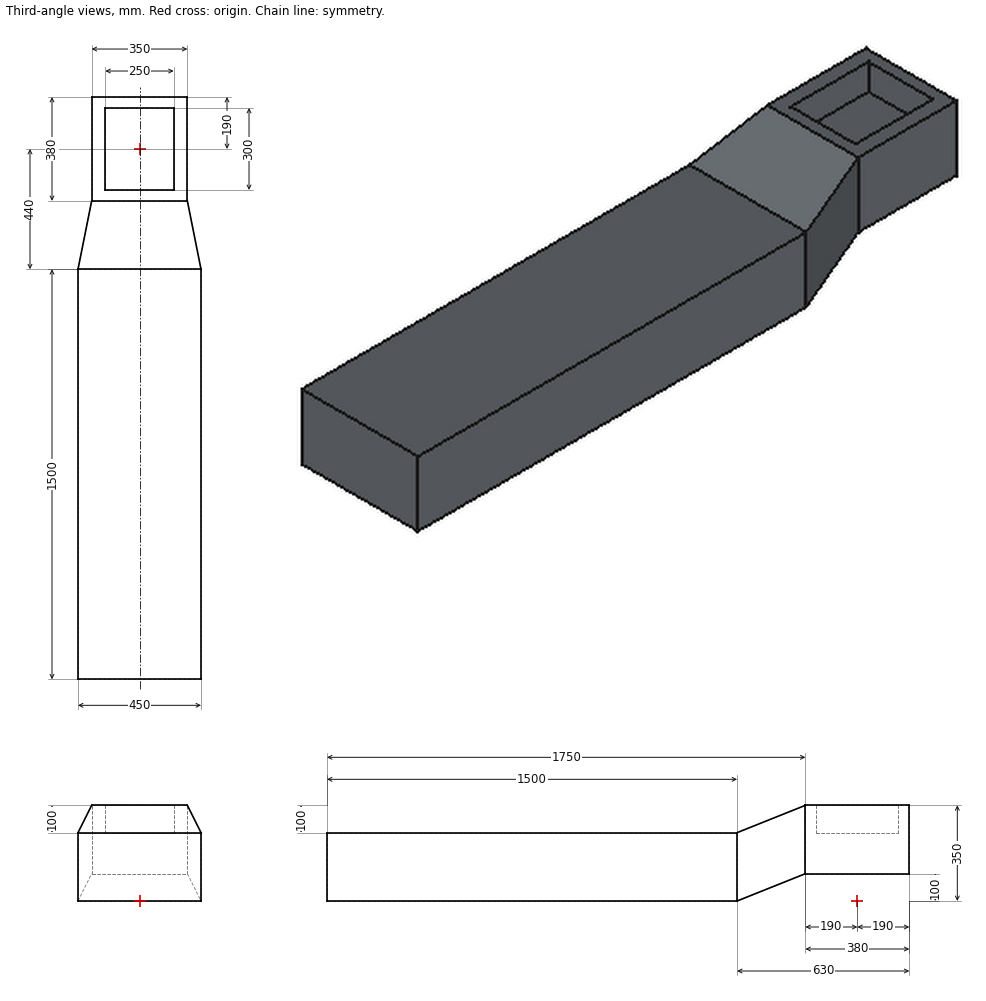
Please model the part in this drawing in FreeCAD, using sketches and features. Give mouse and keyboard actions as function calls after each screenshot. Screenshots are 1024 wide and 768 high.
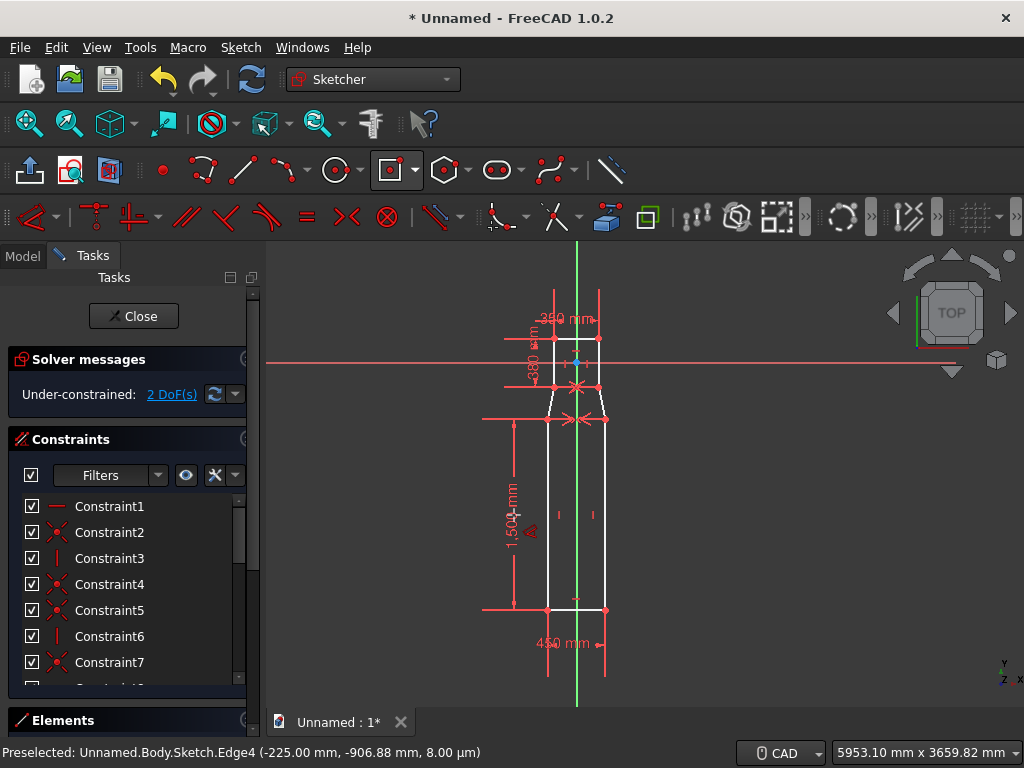
scroll(599, 339, up, 3)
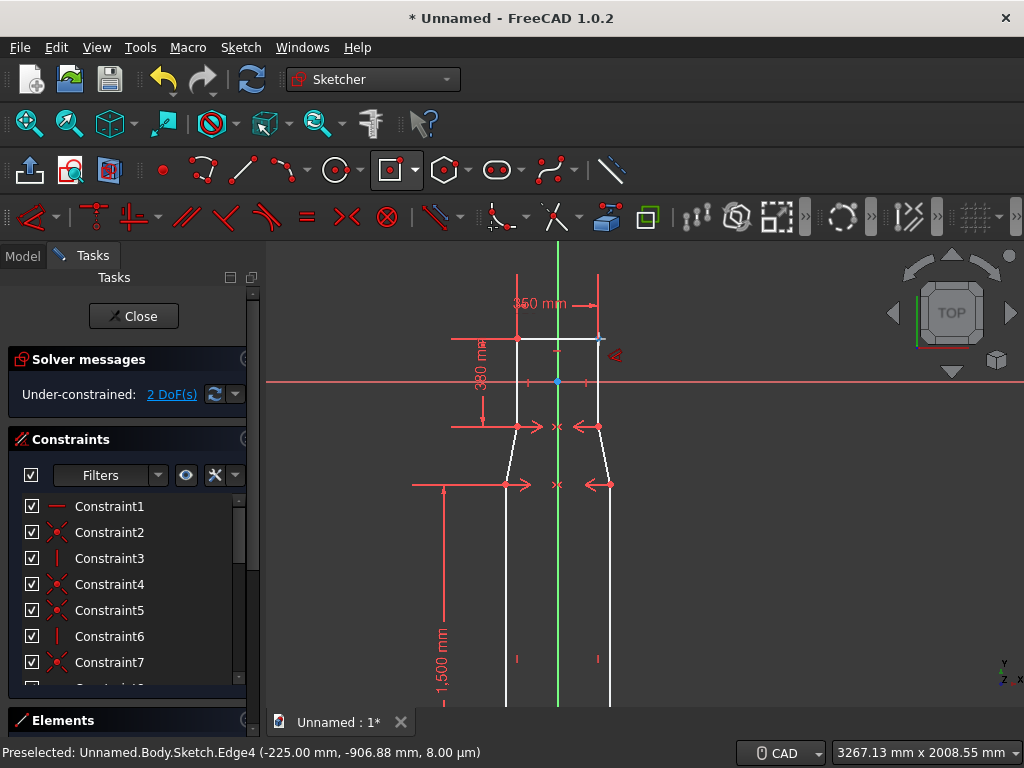
click(598, 339)
click(632, 360)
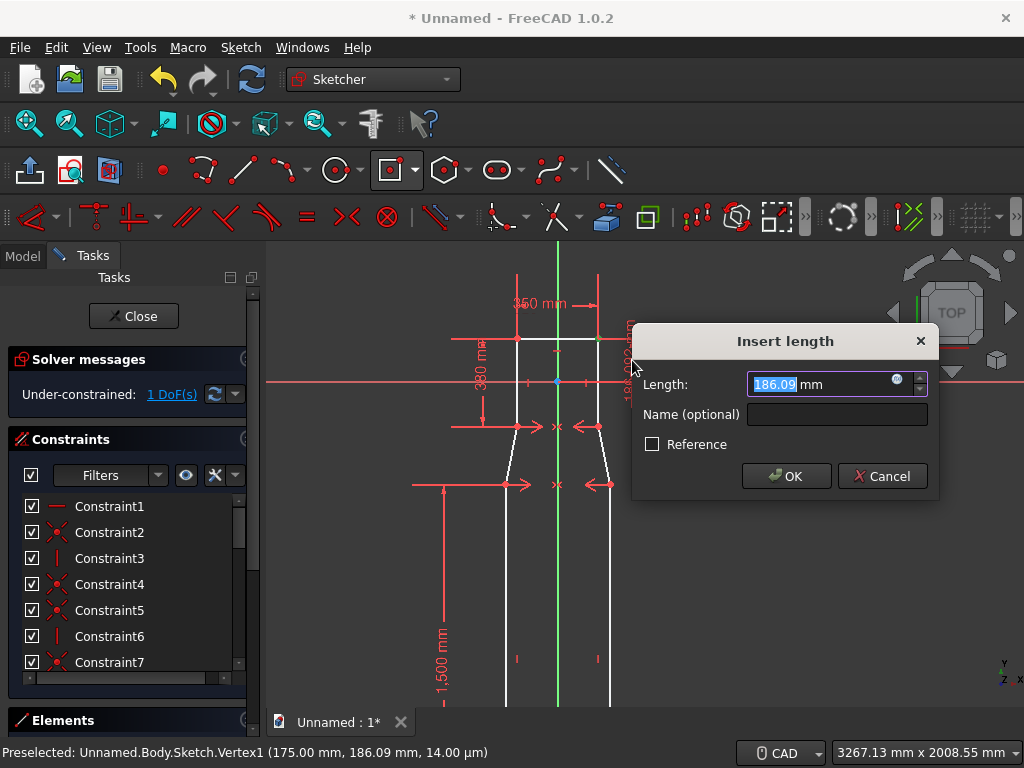
text(190)
key(Return)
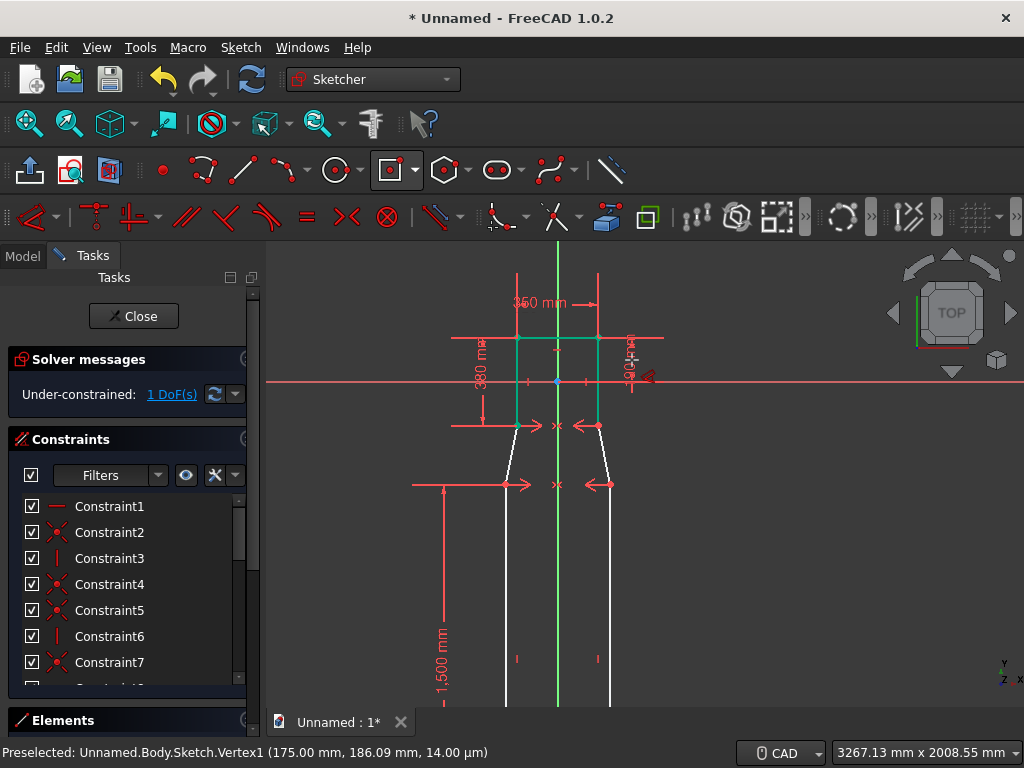
click(506, 485)
click(472, 433)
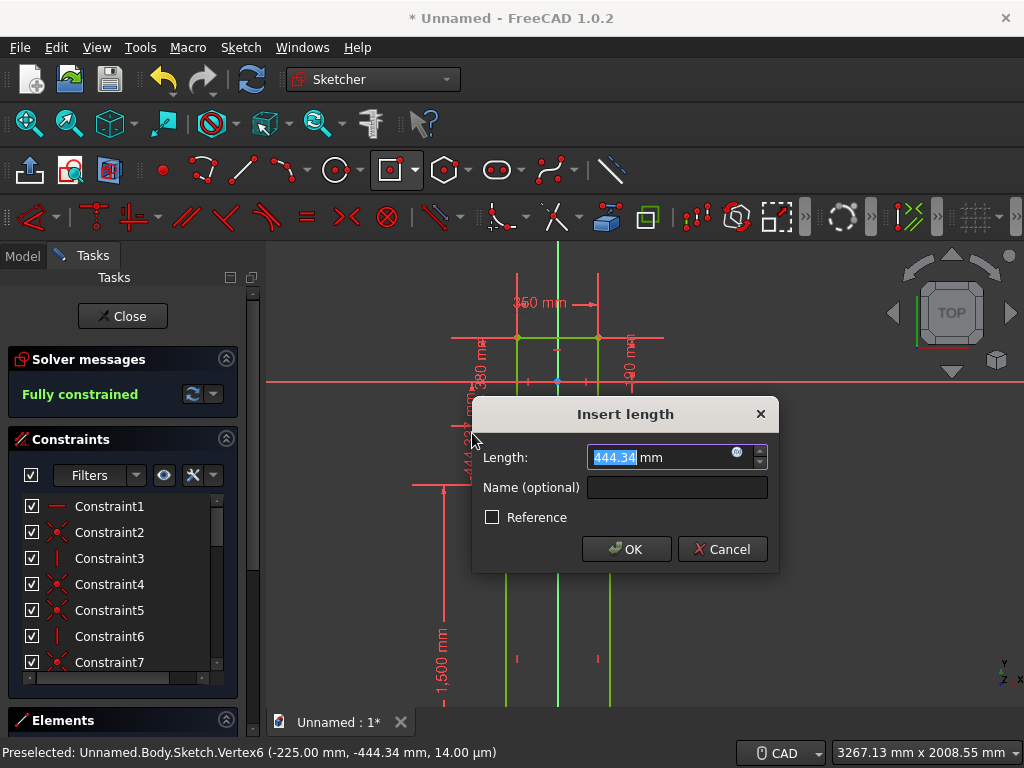
text(440)
key(Return)
key(Escape)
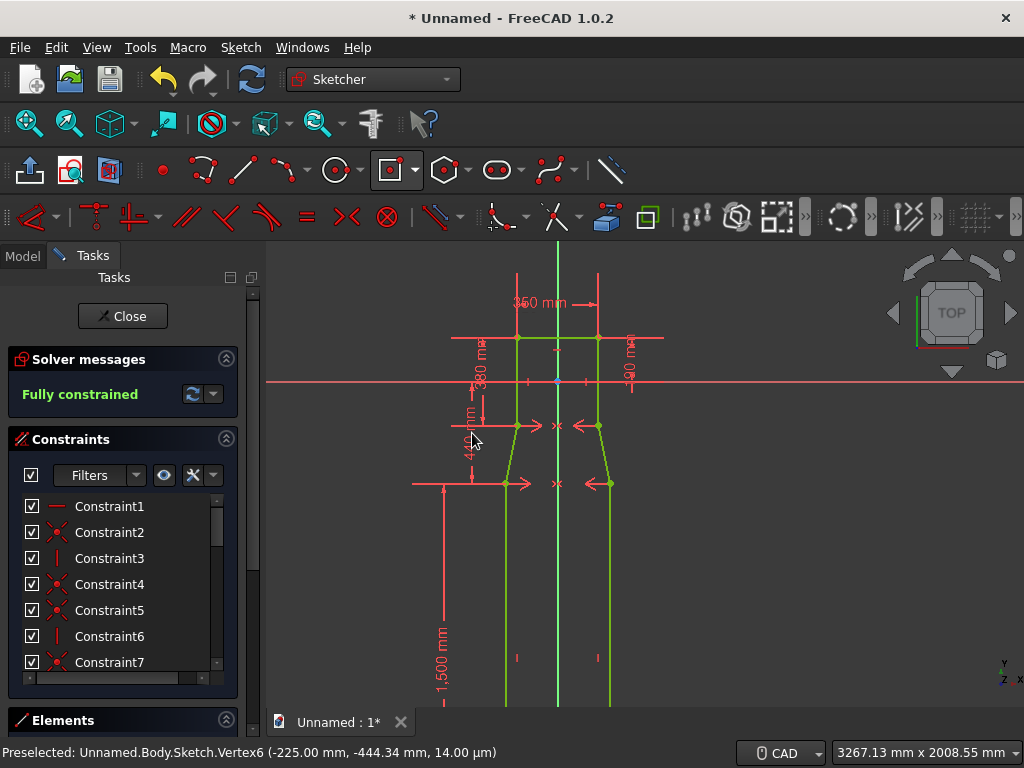
click(123, 316)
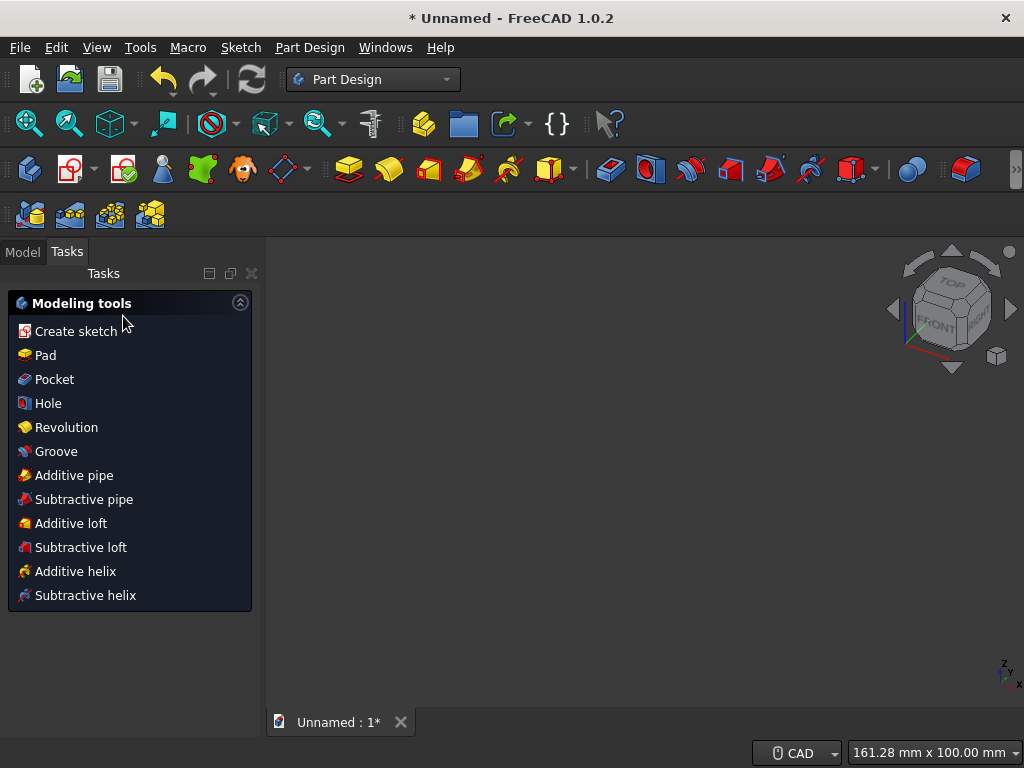
click(350, 170)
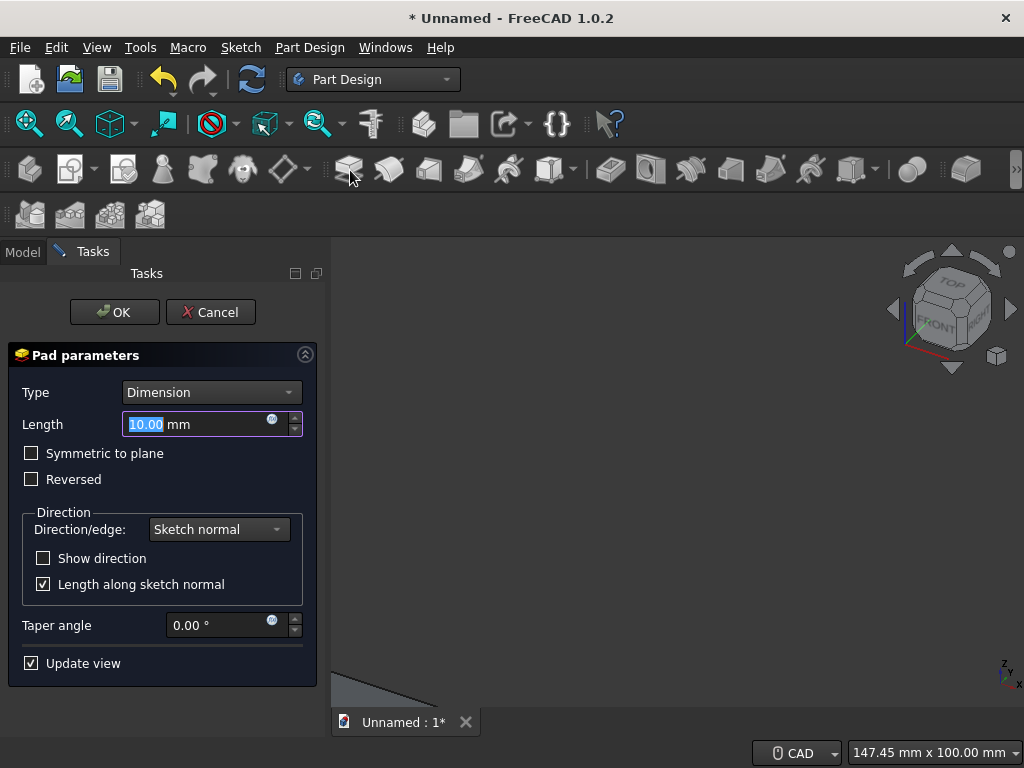
text(350)
key(Tab)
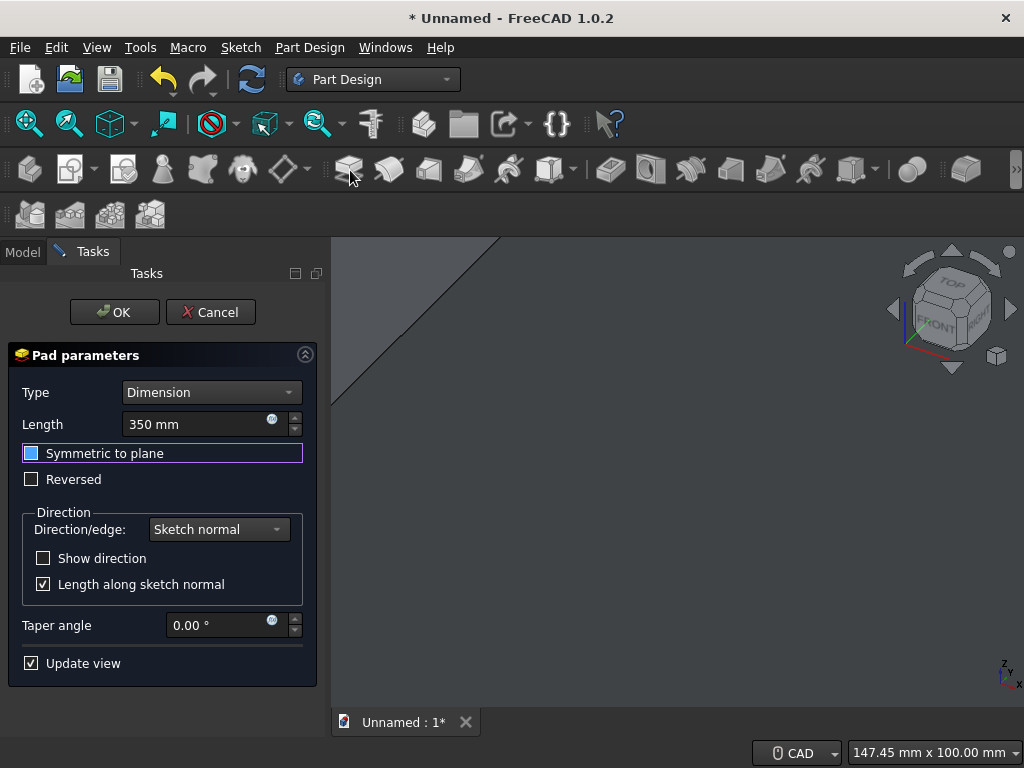
click(115, 312)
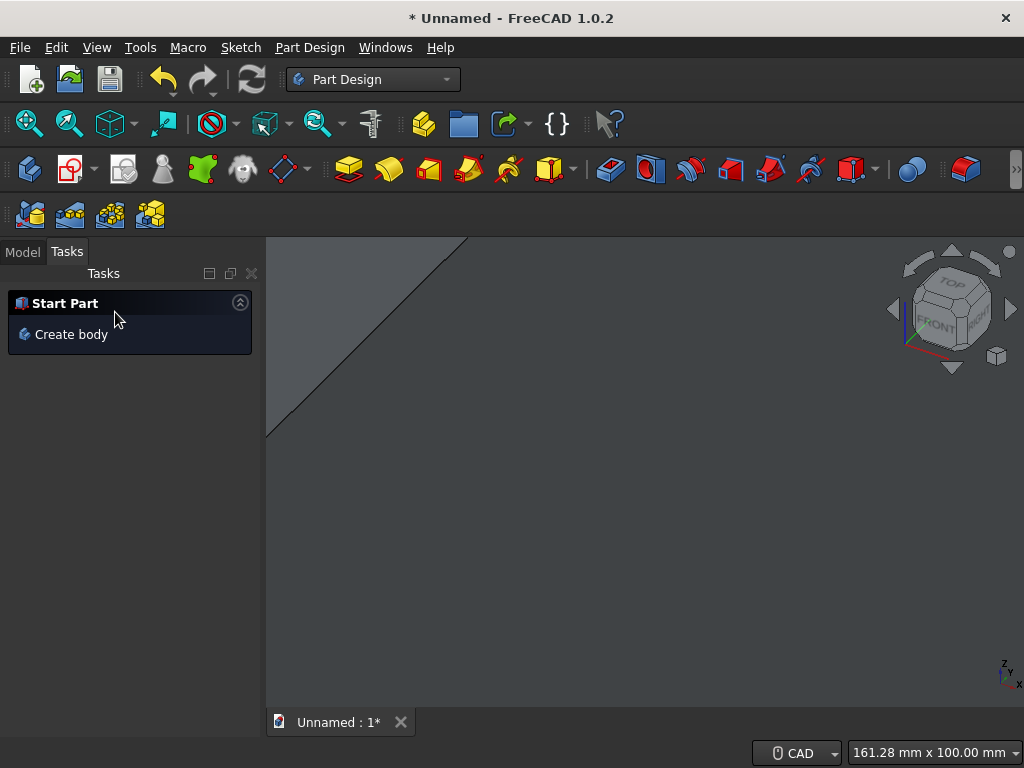
click(30, 124)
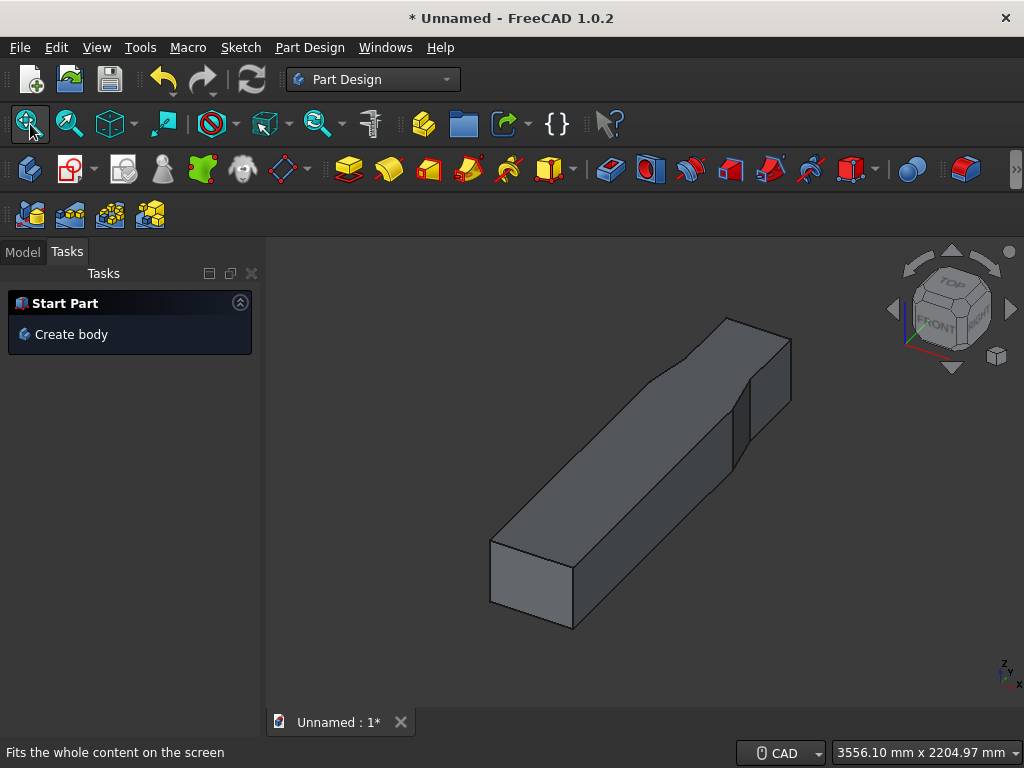
key(6)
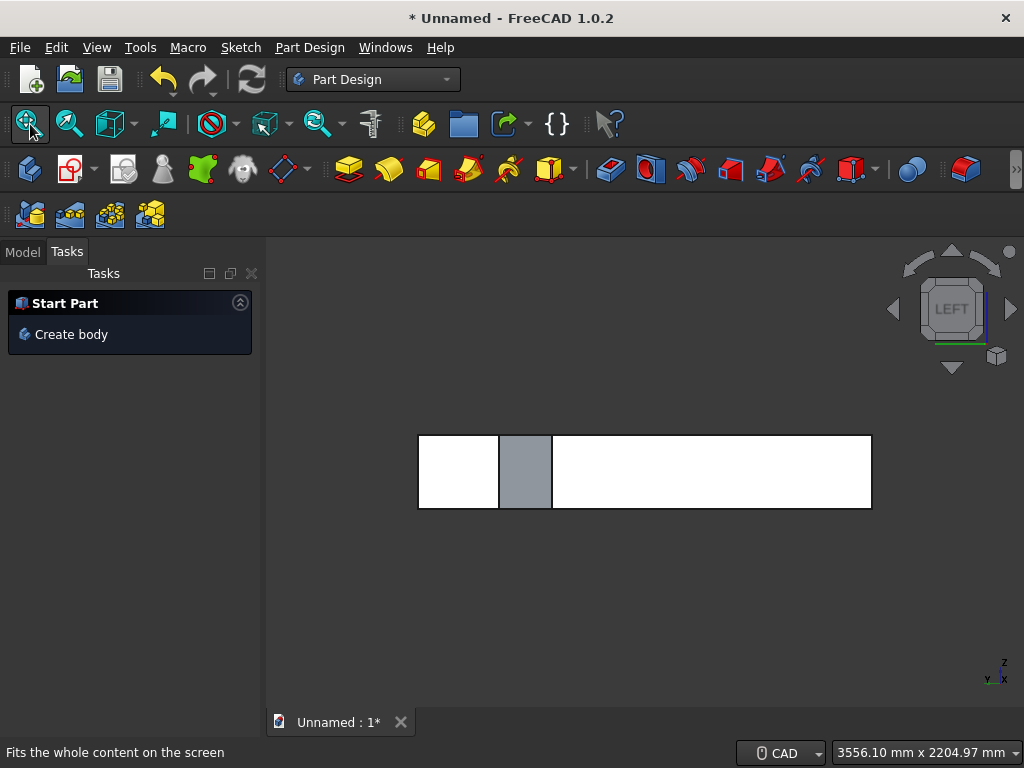
click(621, 471)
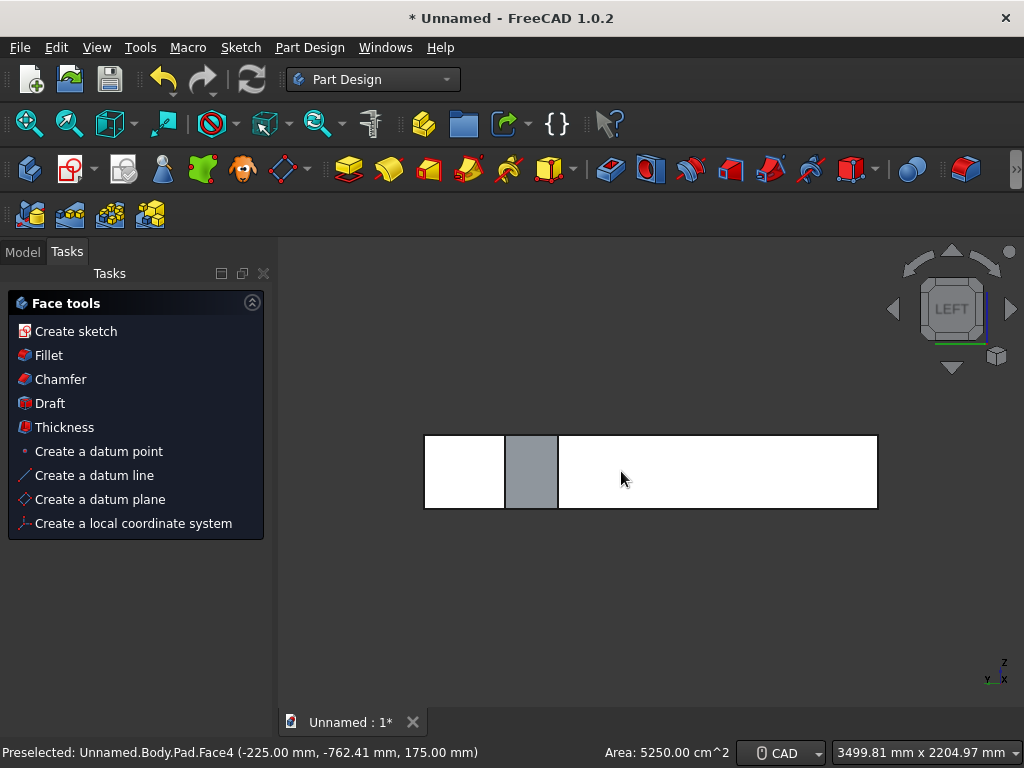
click(70, 170)